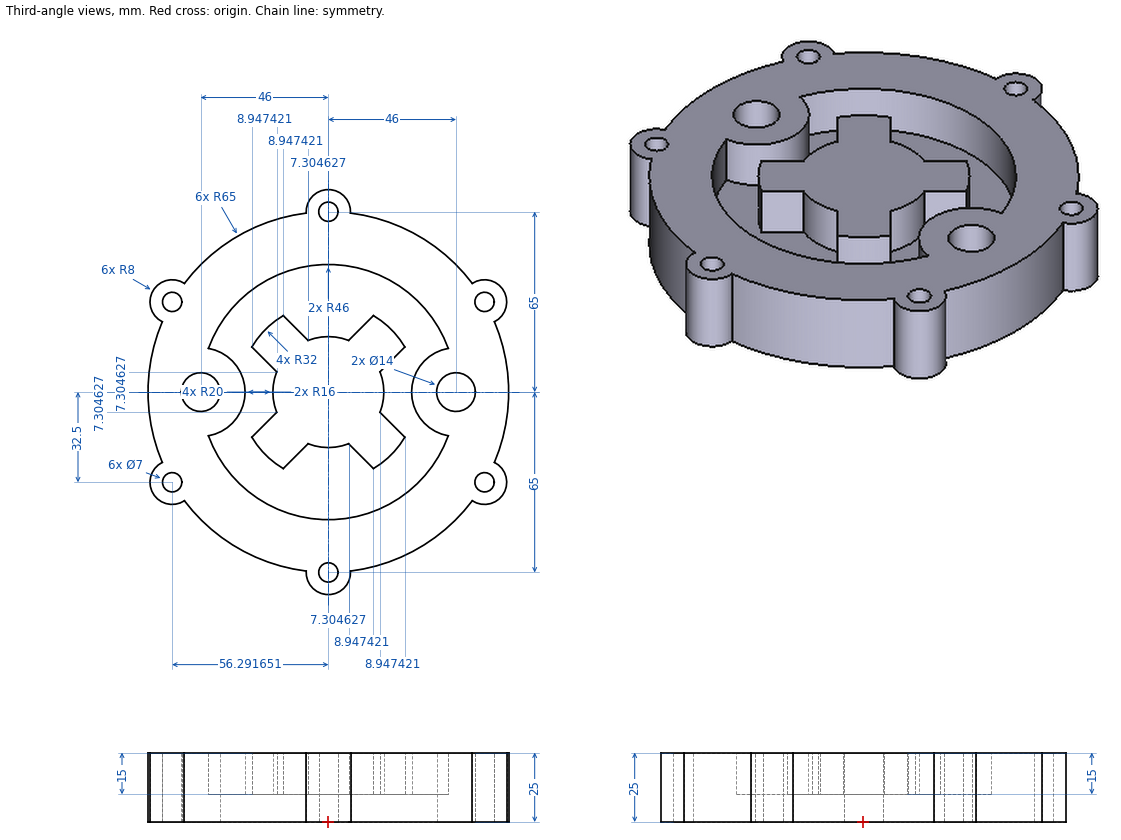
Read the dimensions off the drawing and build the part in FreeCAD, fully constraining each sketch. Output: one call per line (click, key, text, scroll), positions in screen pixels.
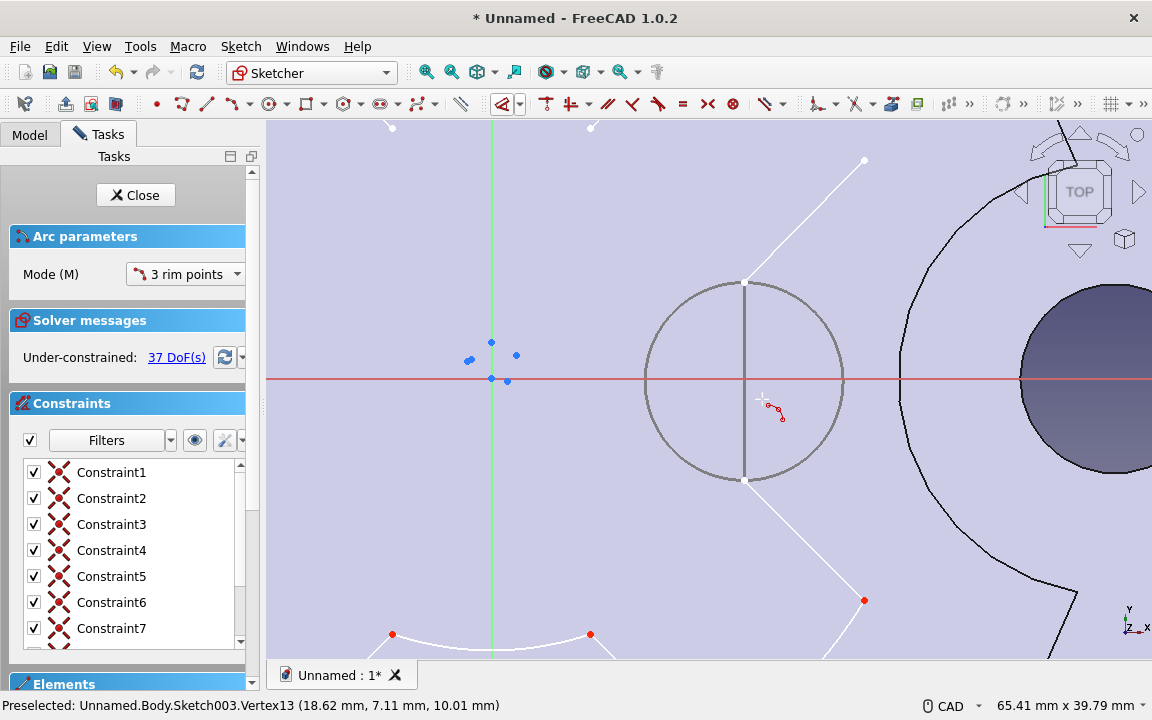
click(762, 399)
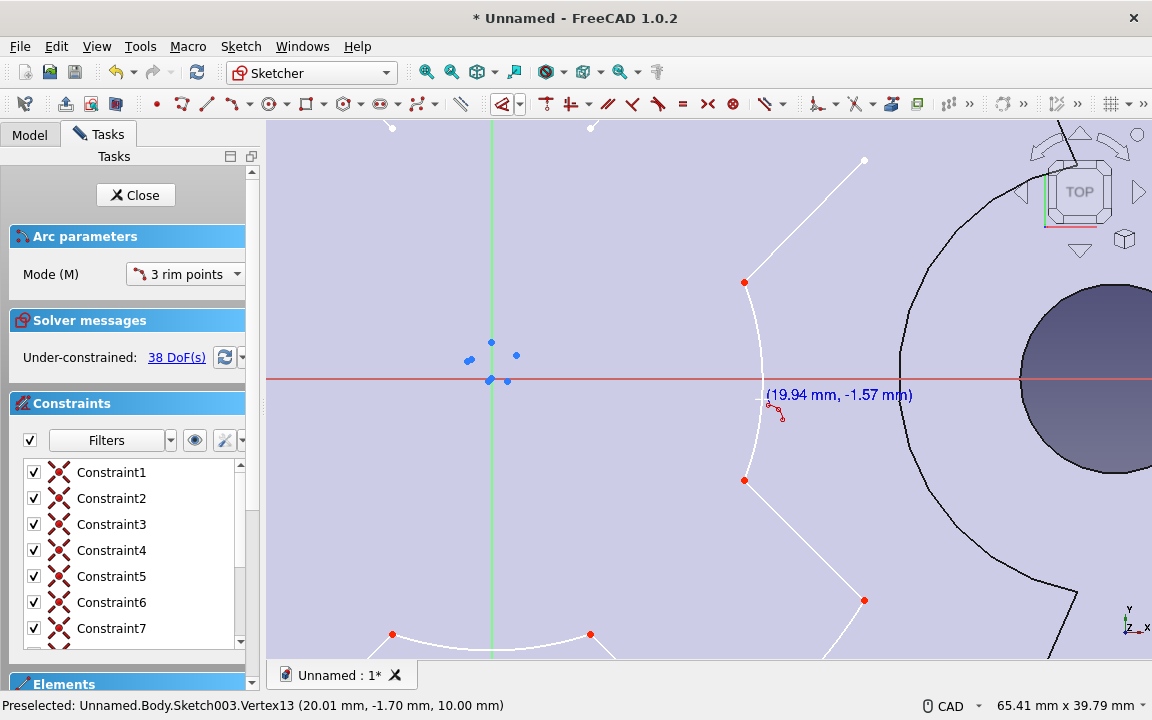
click(864, 160)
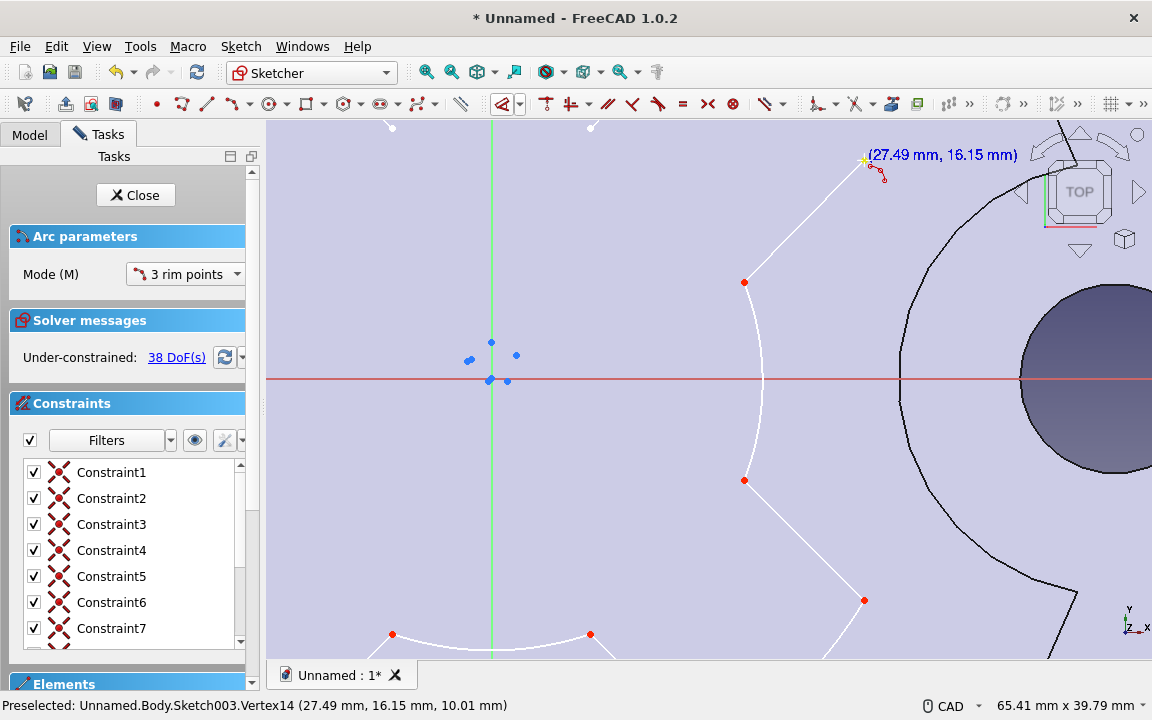
scroll(762, 398, down, 4)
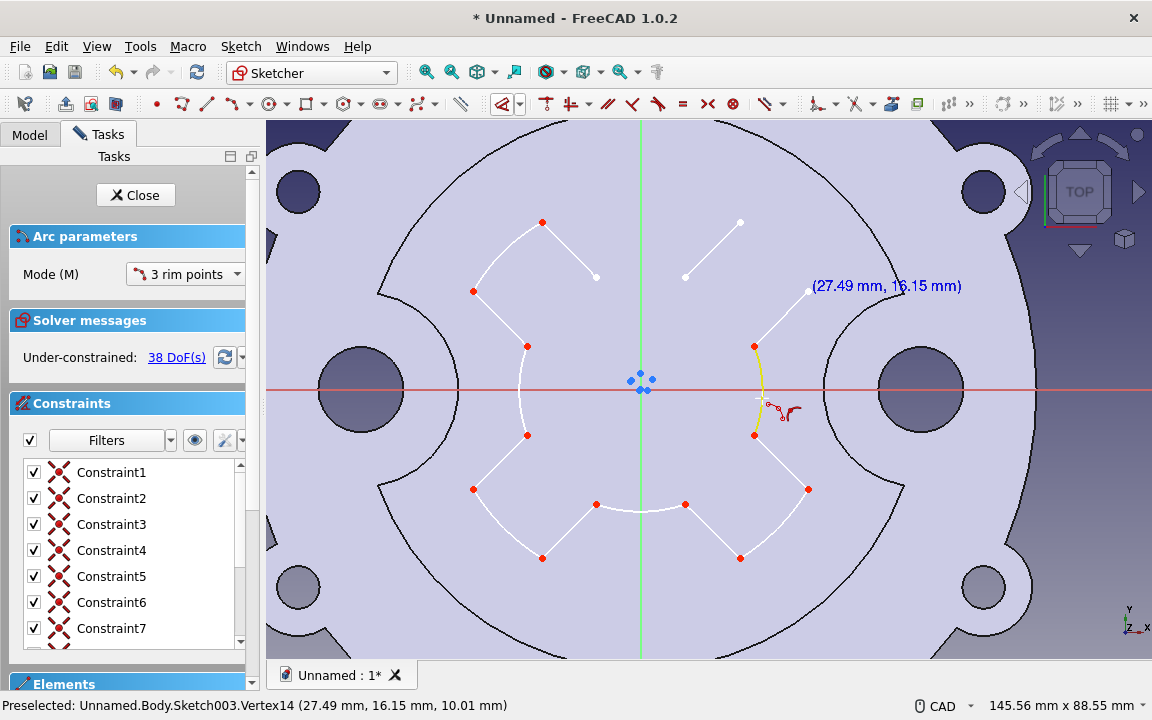
click(740, 222)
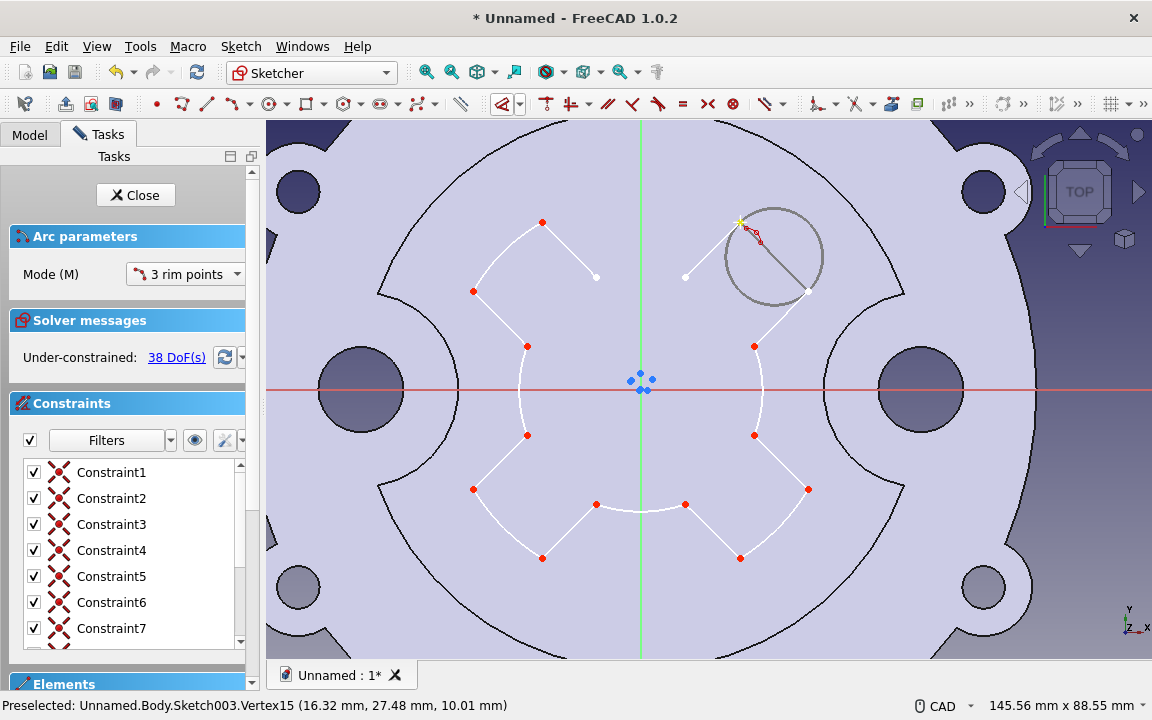
scroll(779, 252, up, 5)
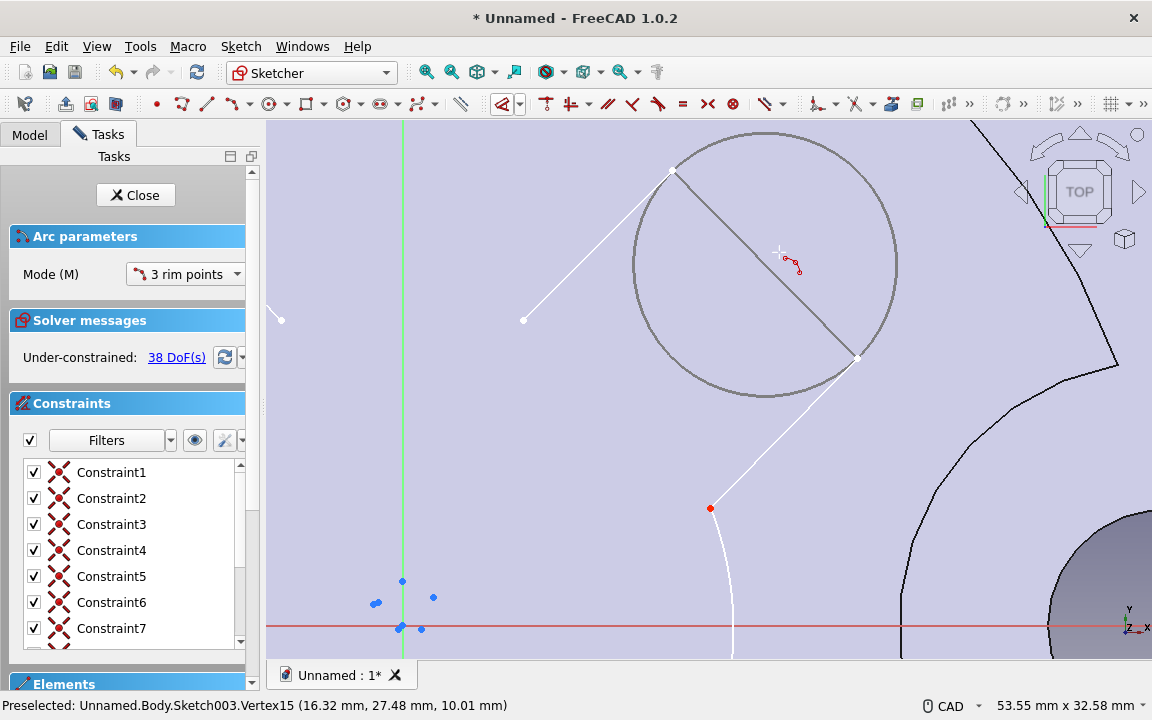
click(777, 251)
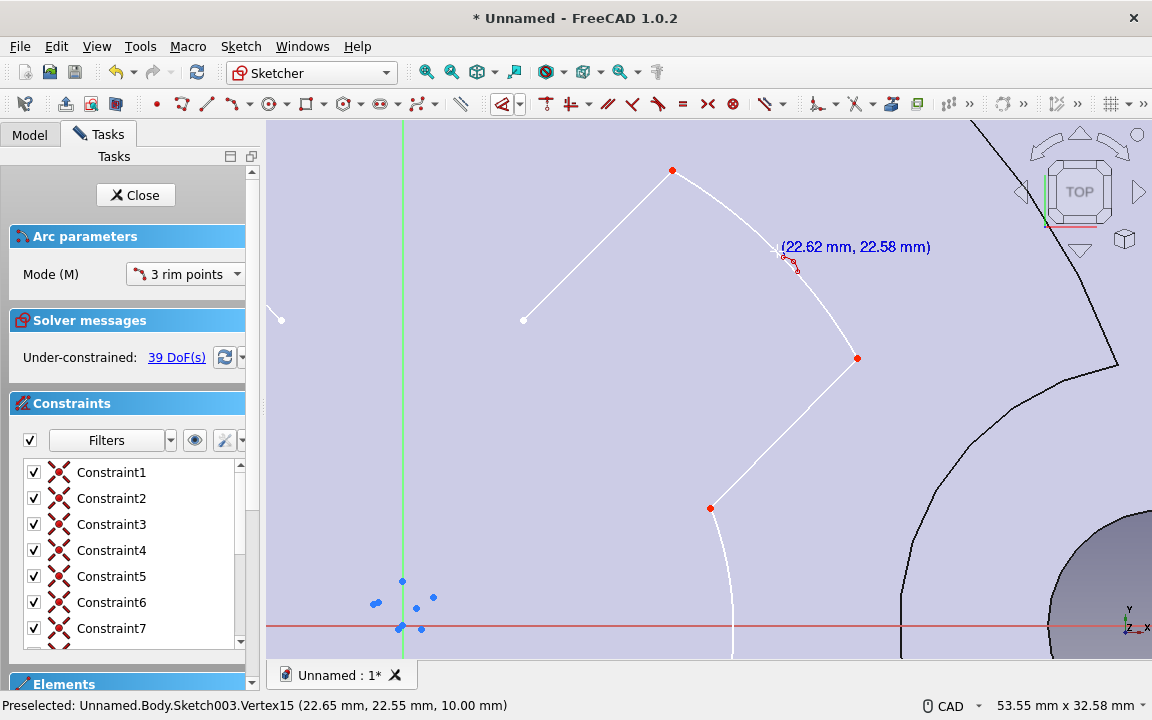
click(523, 320)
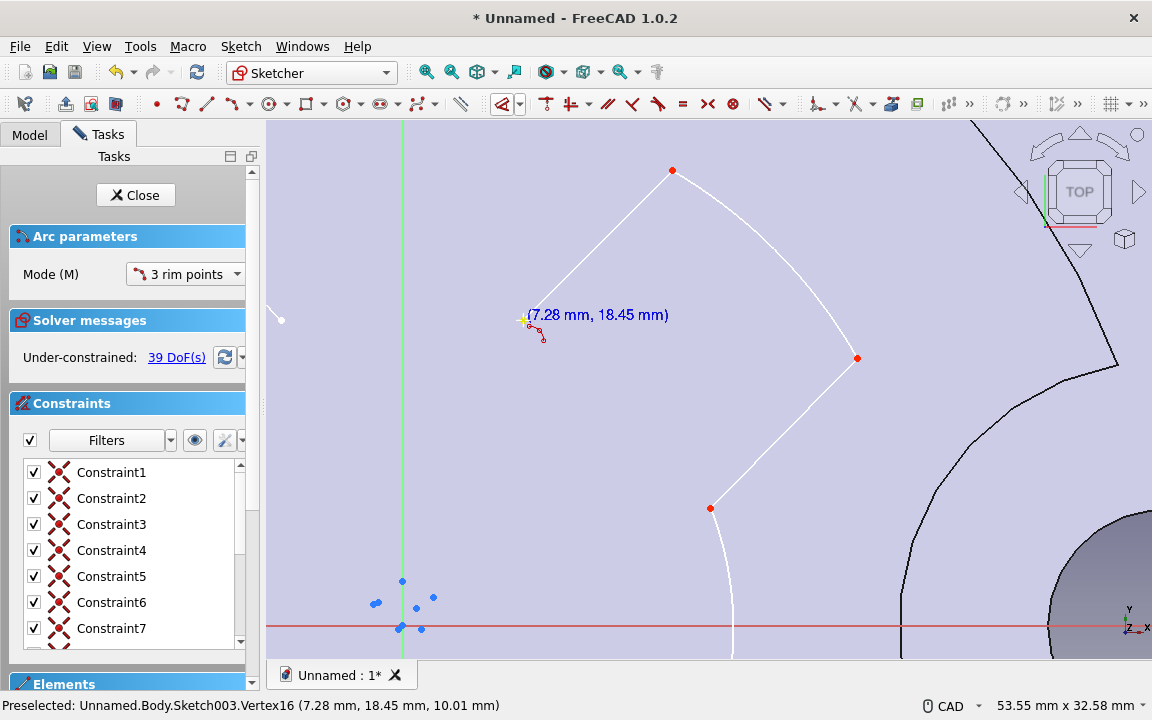
scroll(779, 252, down, 5)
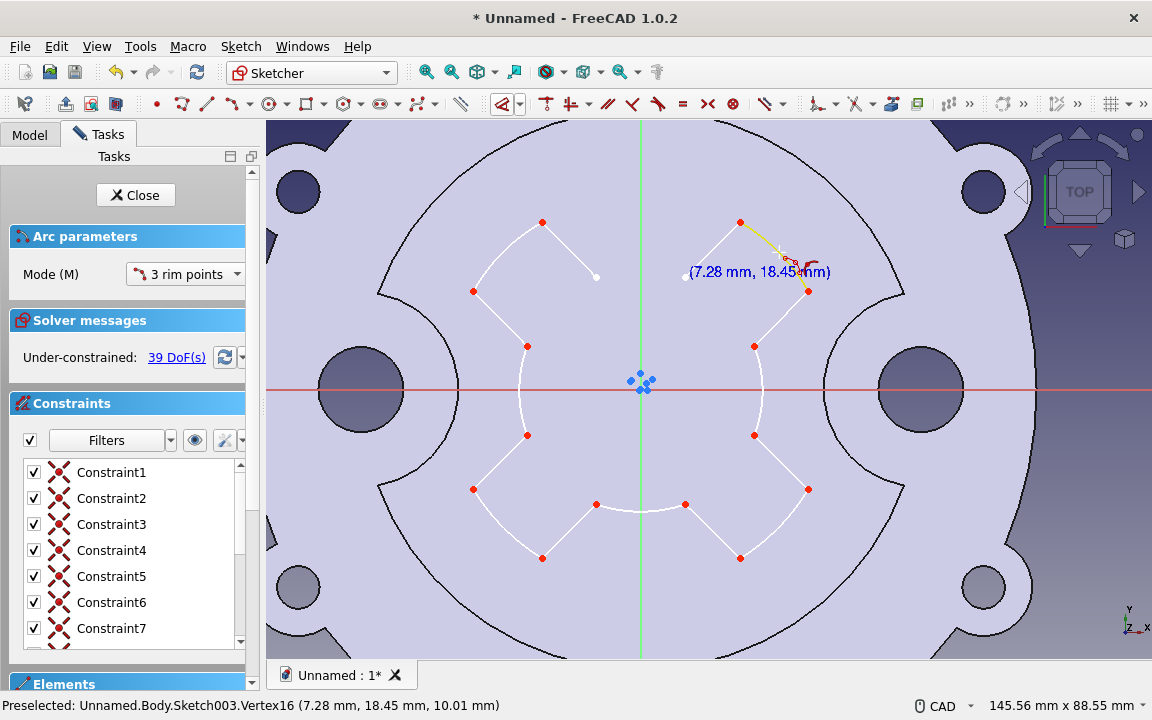
click(596, 277)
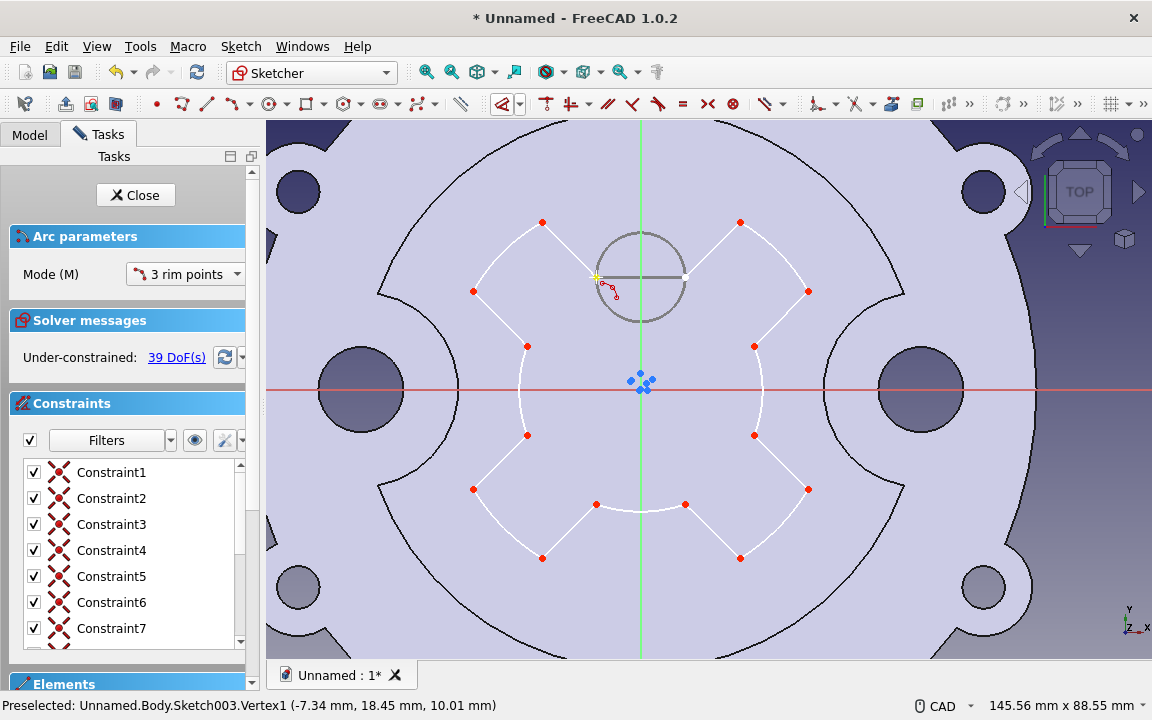
scroll(650, 268, up, 4)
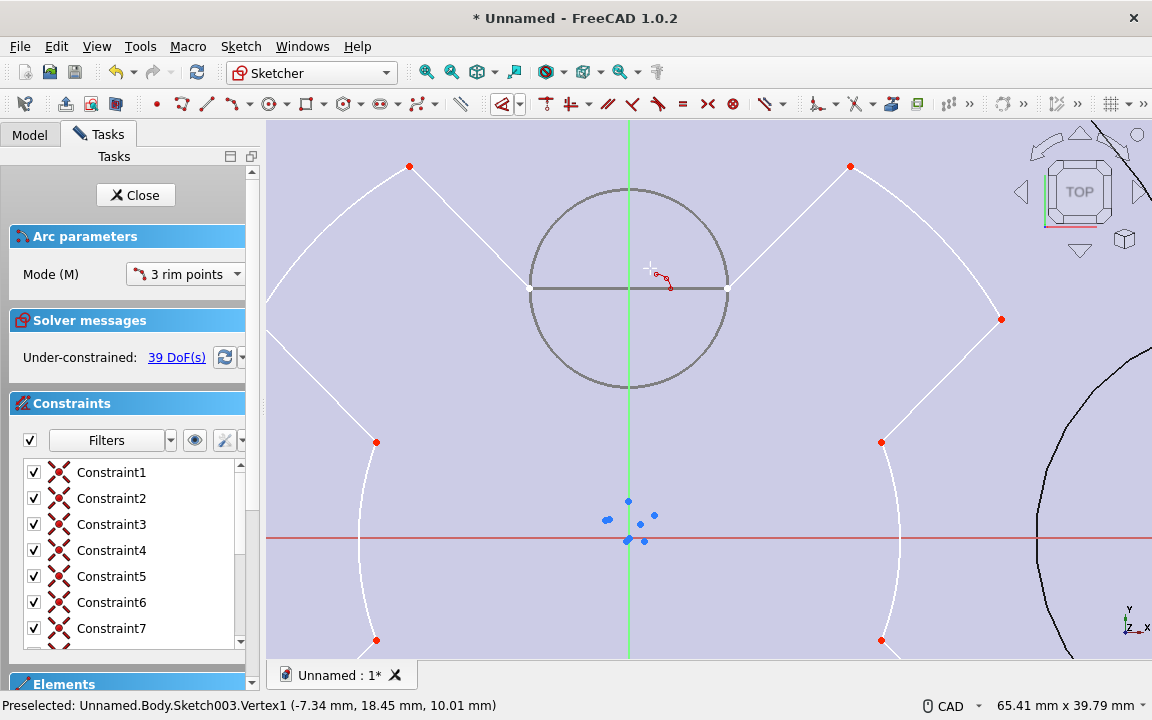
click(650, 268)
key(Escape)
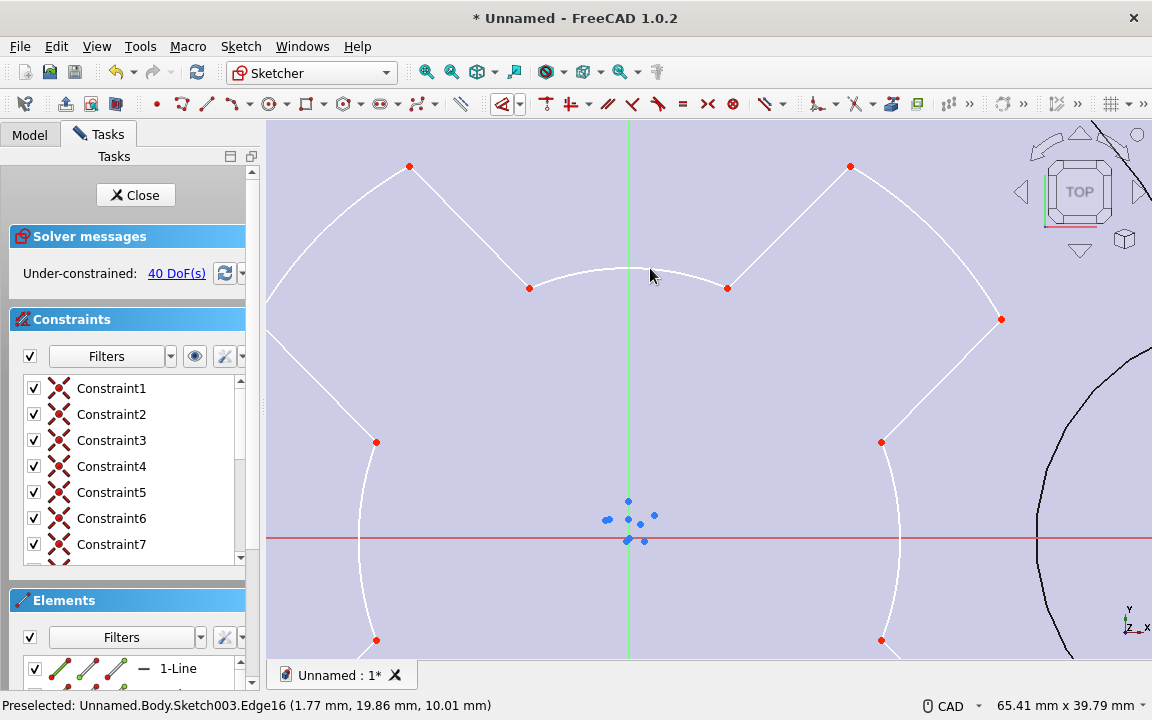
click(355, 203)